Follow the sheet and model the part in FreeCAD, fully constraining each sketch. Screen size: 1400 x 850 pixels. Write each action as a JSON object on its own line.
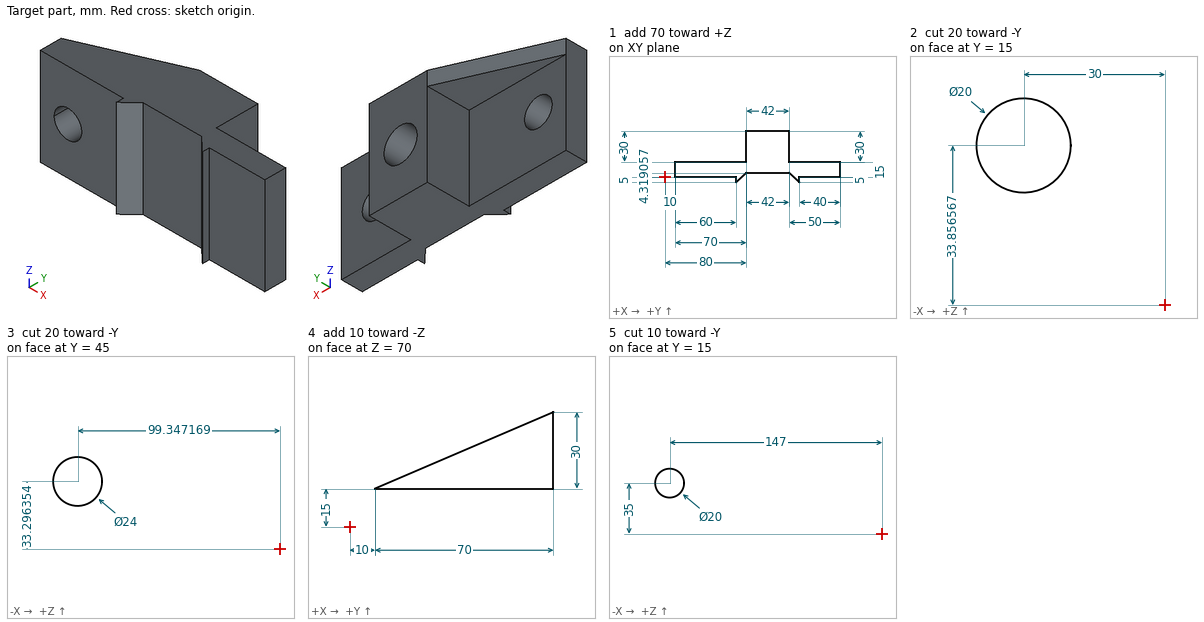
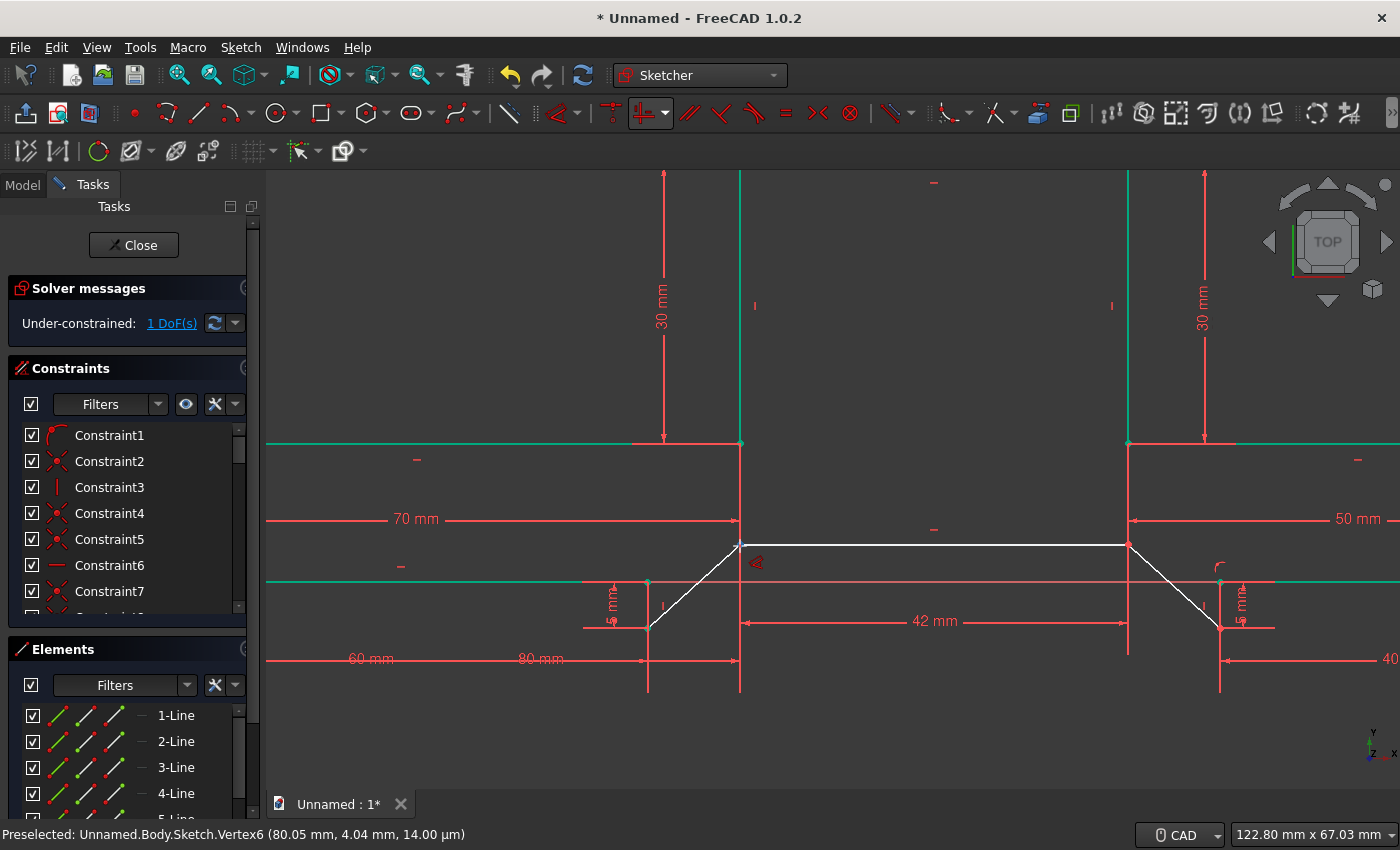
{"action": "left_click", "coordinate": [740, 545]}
{"action": "left_click", "coordinate": [774, 564]}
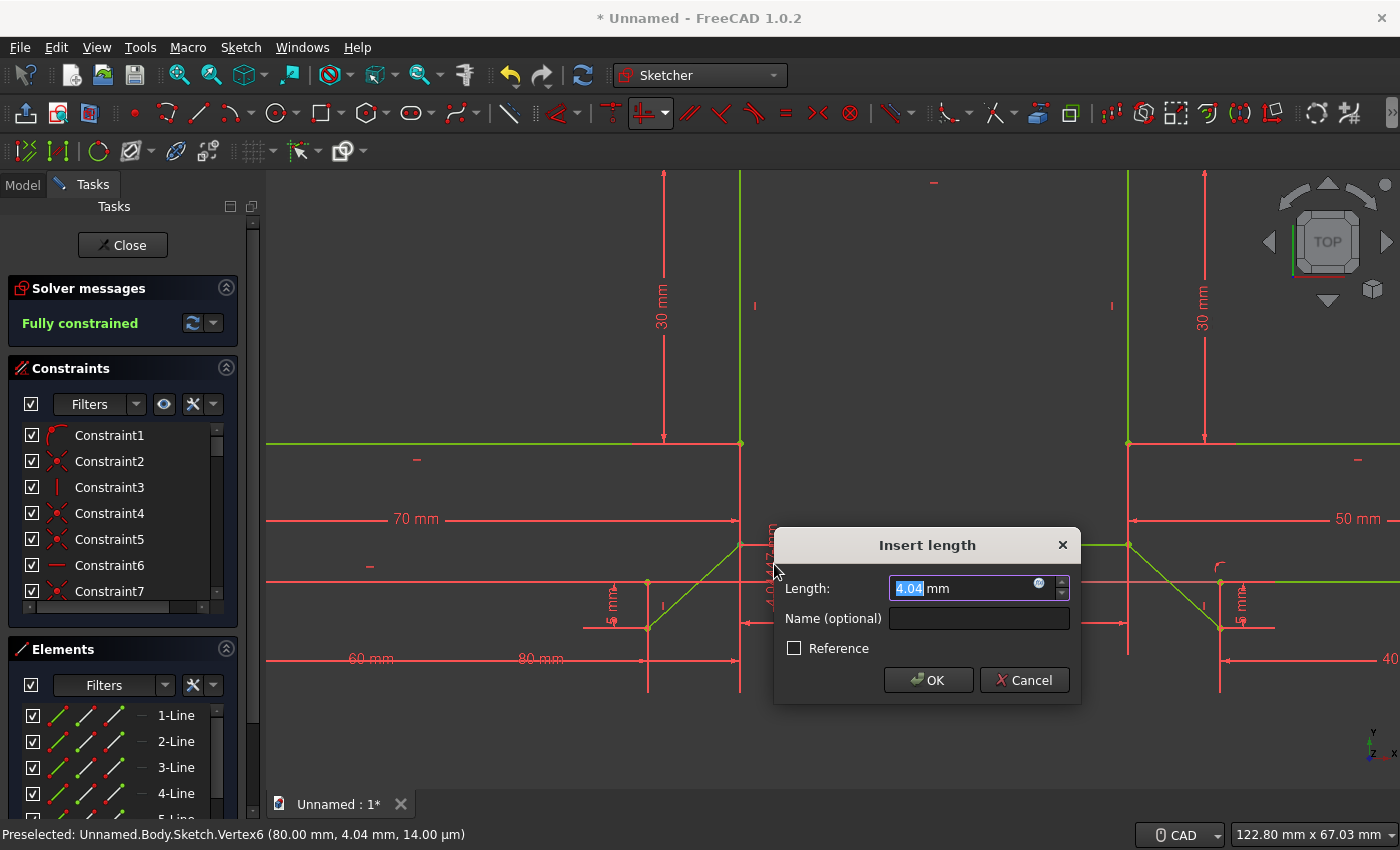
{"action": "type", "text": "4.319057"}
{"action": "key", "text": "Return"}
{"action": "key", "text": "Escape"}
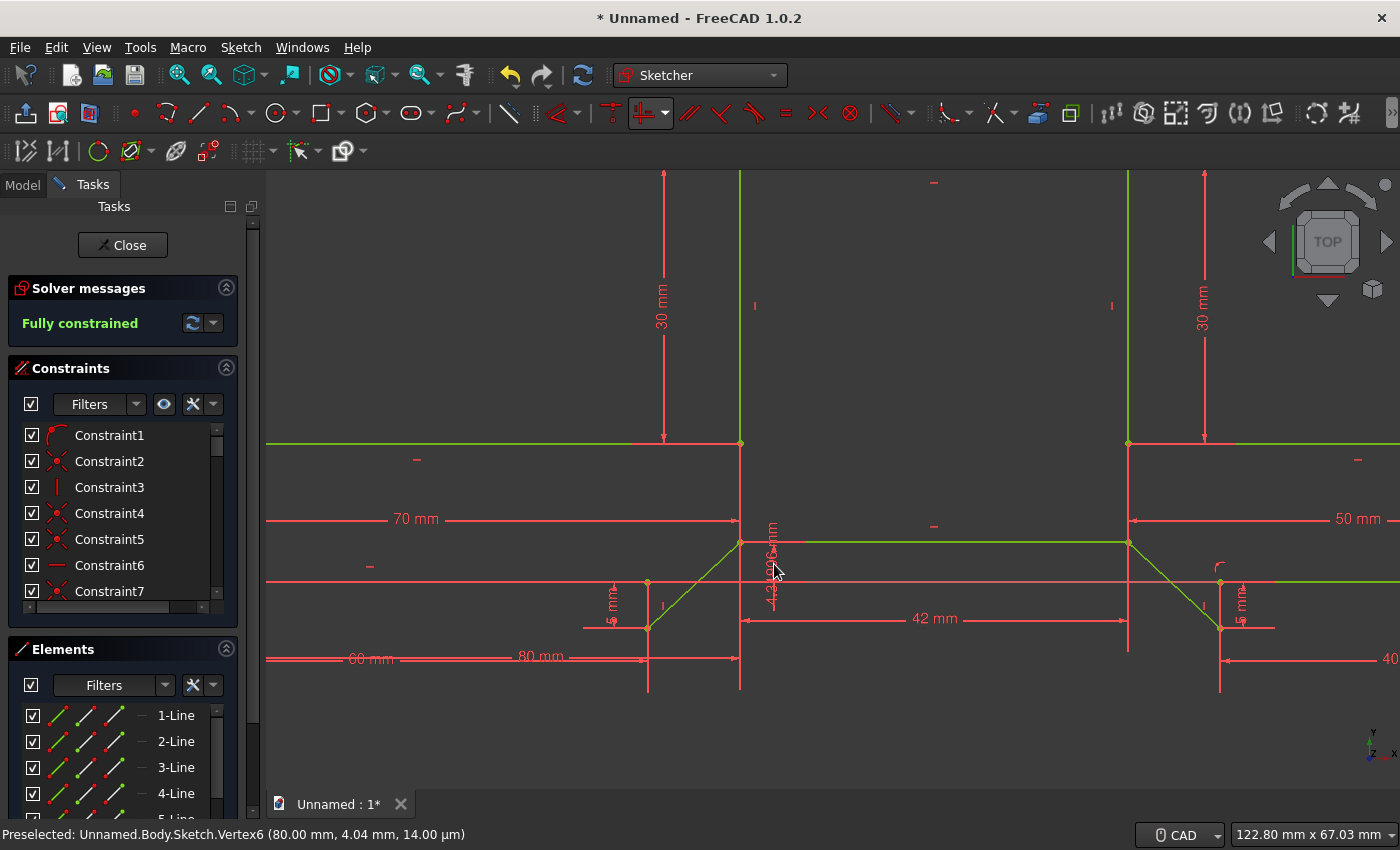
{"action": "left_click", "coordinate": [123, 245]}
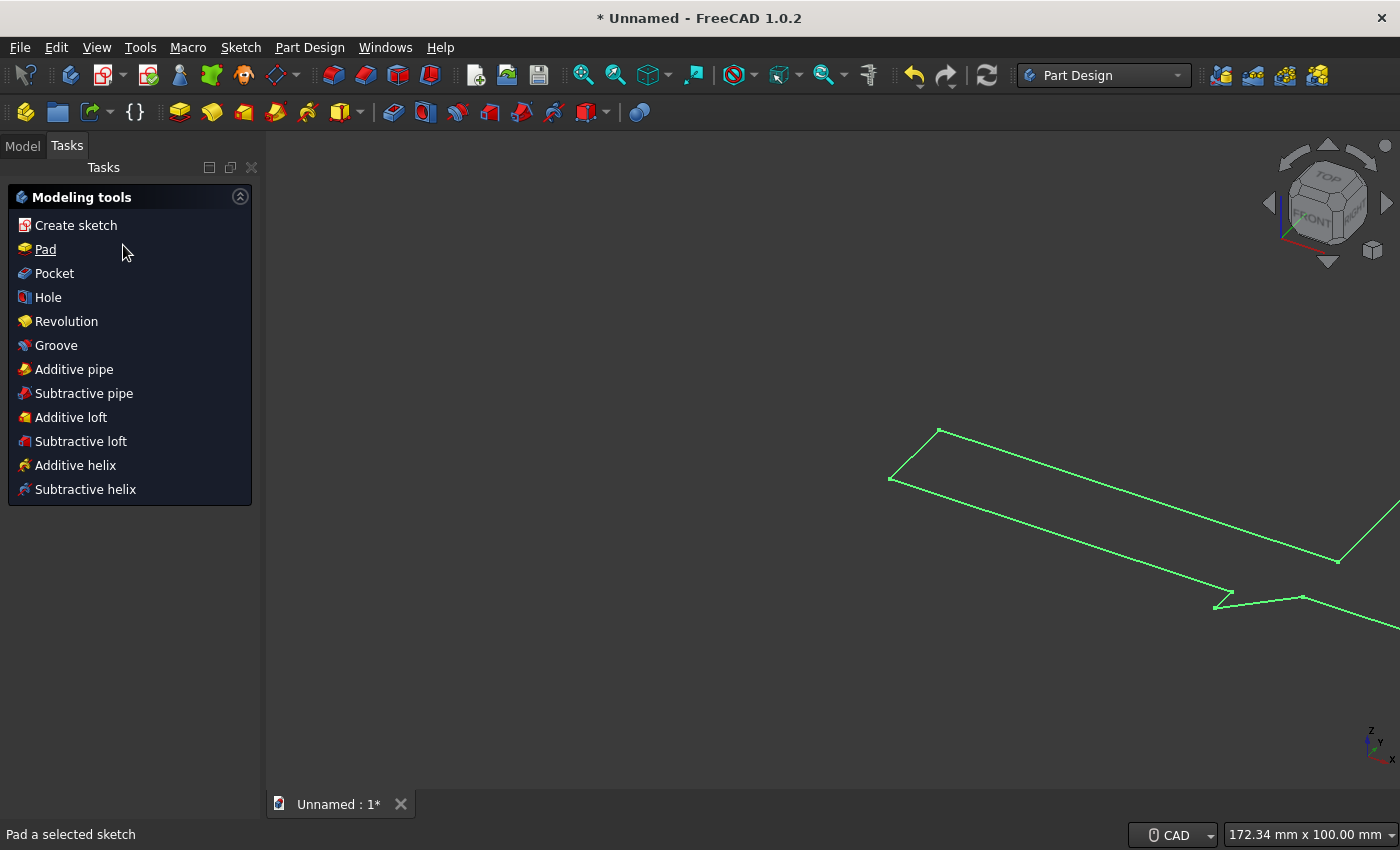
{"action": "left_click", "coordinate": [180, 112]}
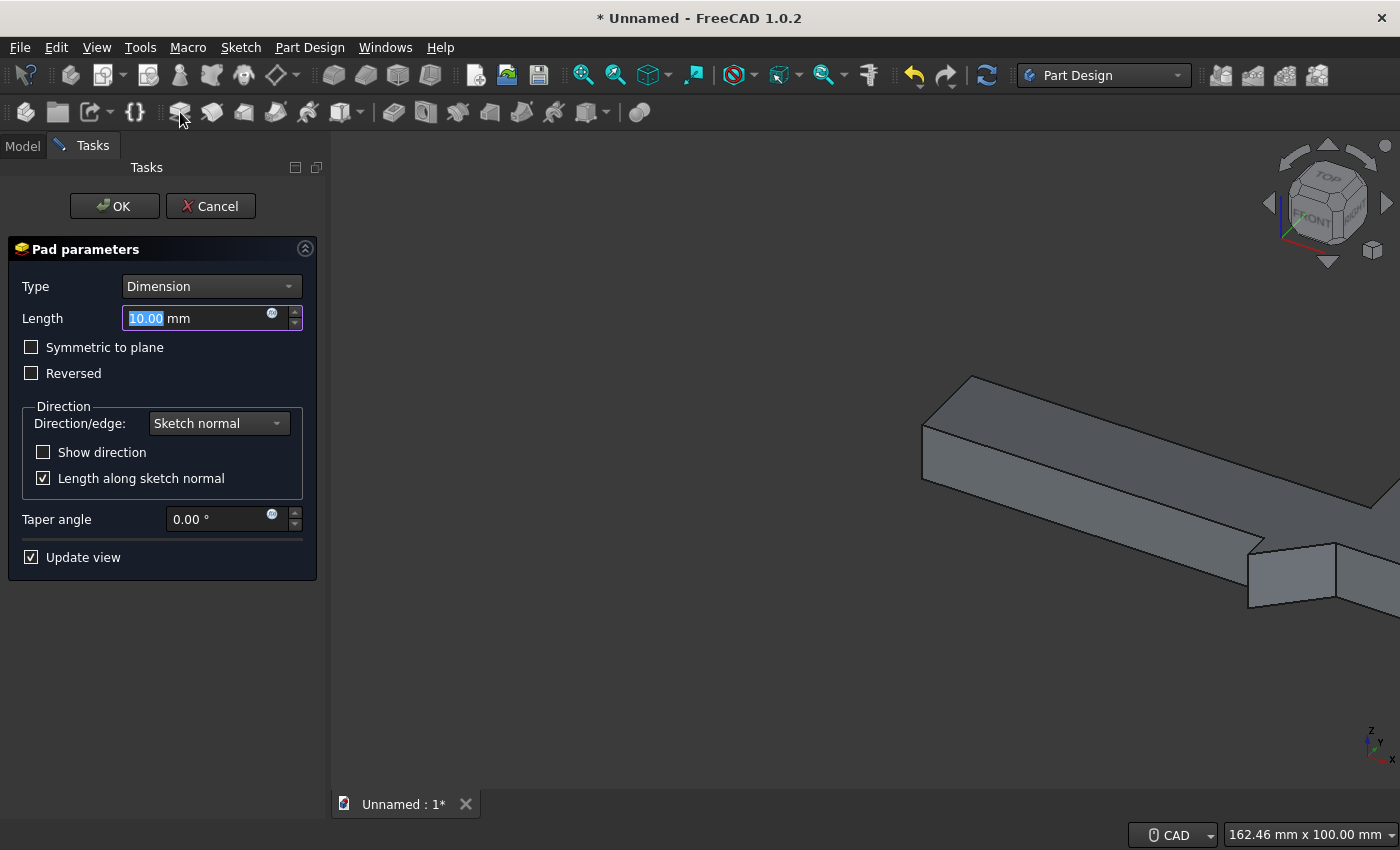
{"action": "type", "text": "70"}
{"action": "key", "text": "Tab"}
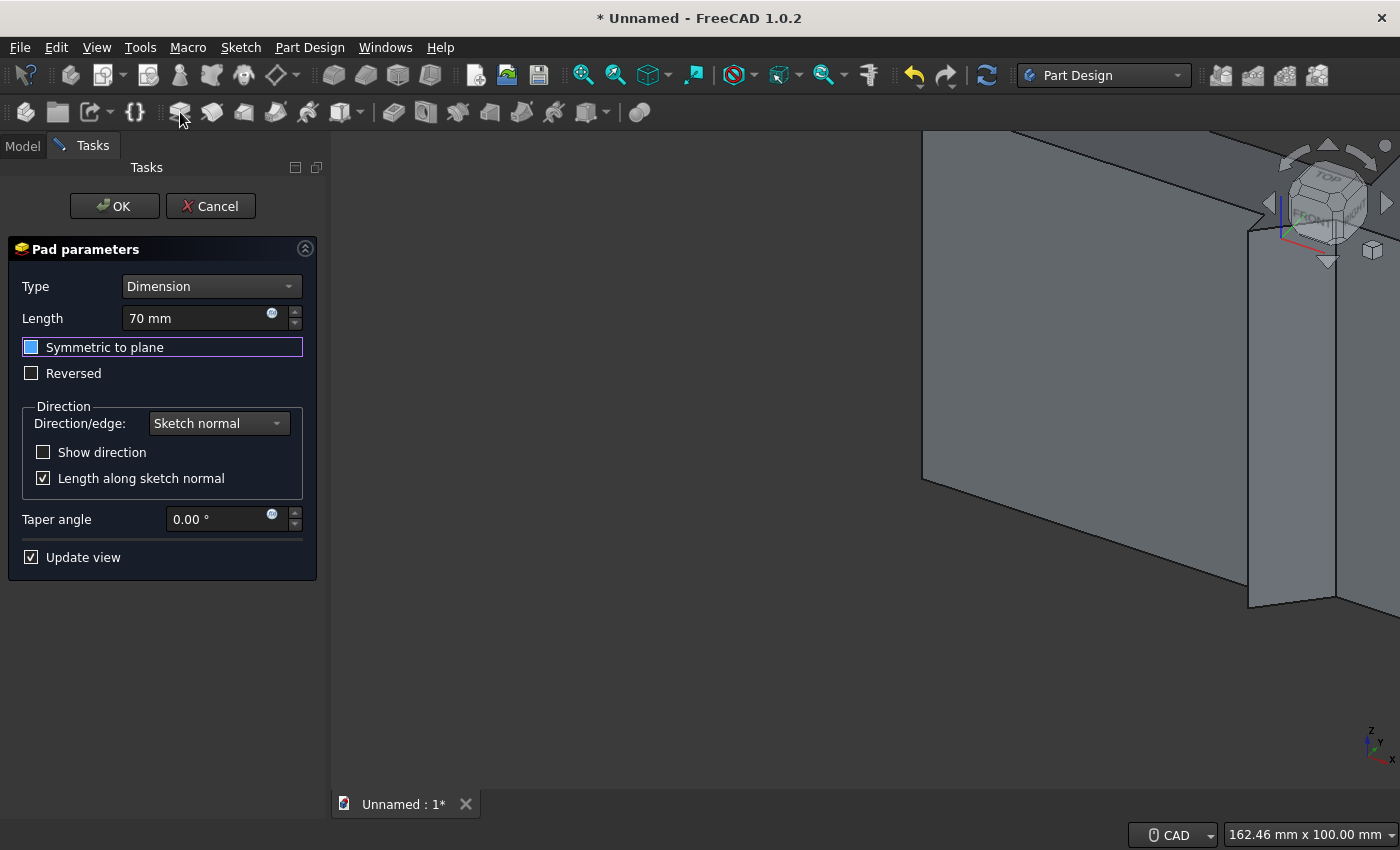
{"action": "left_click", "coordinate": [115, 206]}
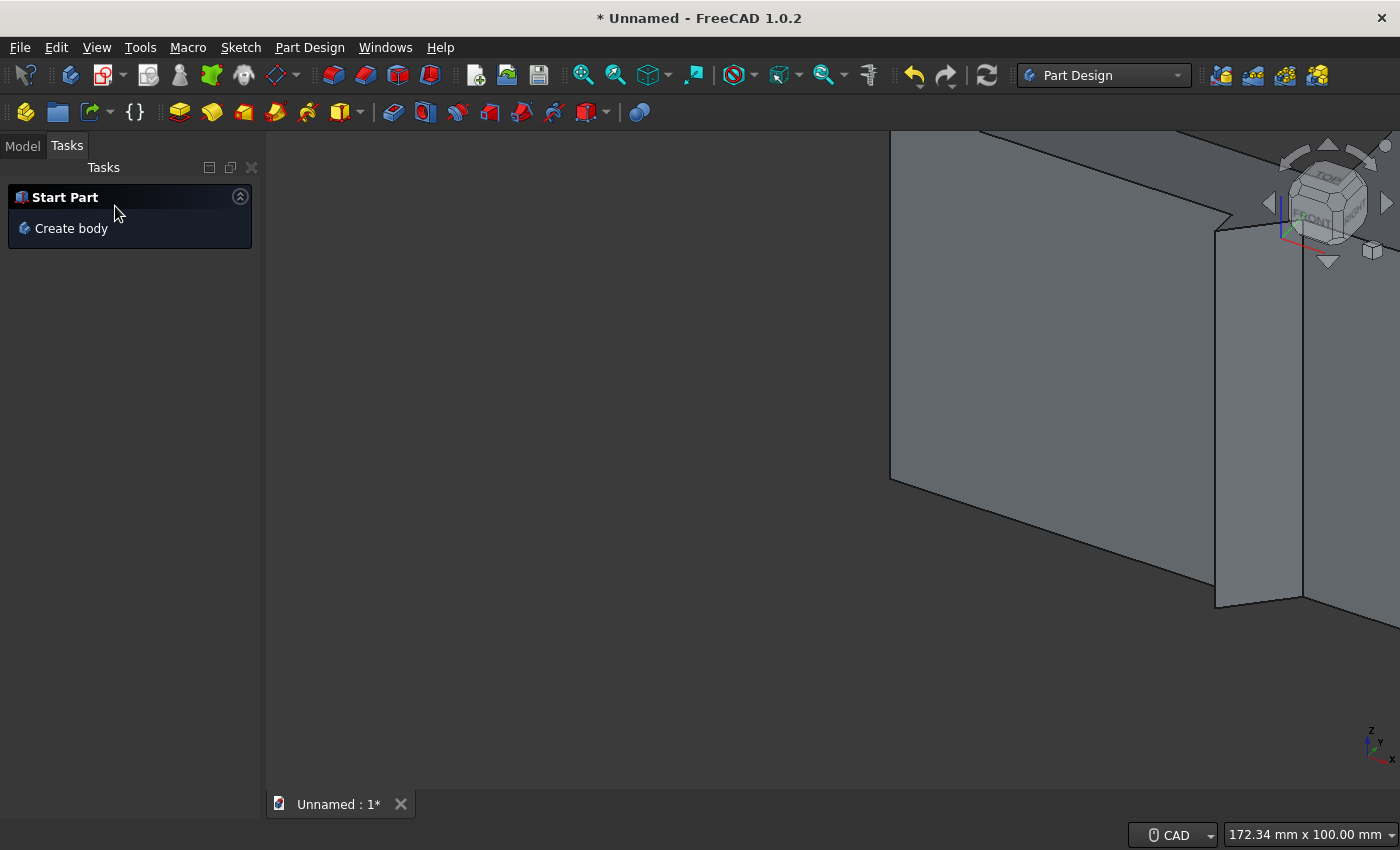
{"action": "left_click", "coordinate": [584, 76]}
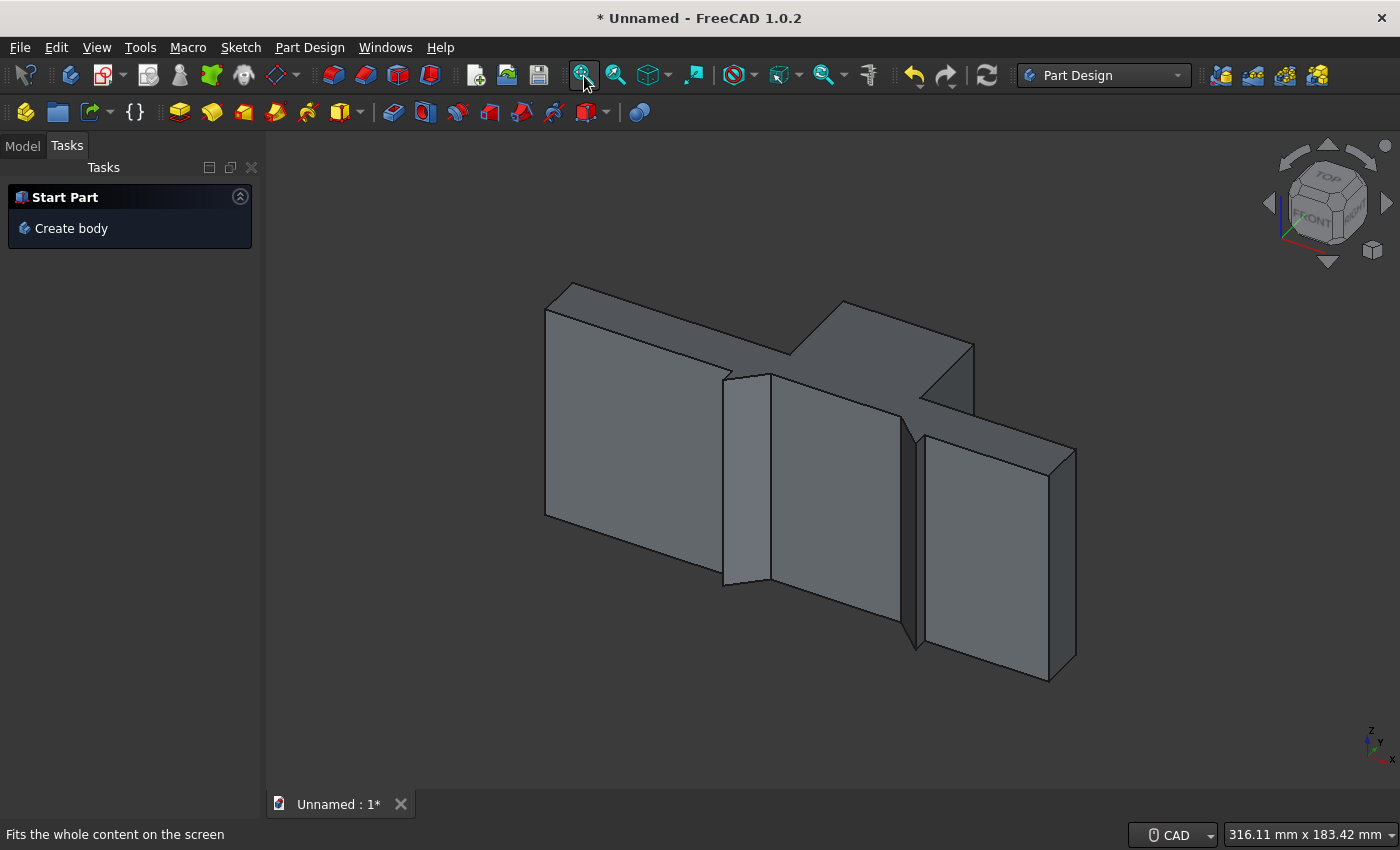
{"action": "key", "text": "4"}